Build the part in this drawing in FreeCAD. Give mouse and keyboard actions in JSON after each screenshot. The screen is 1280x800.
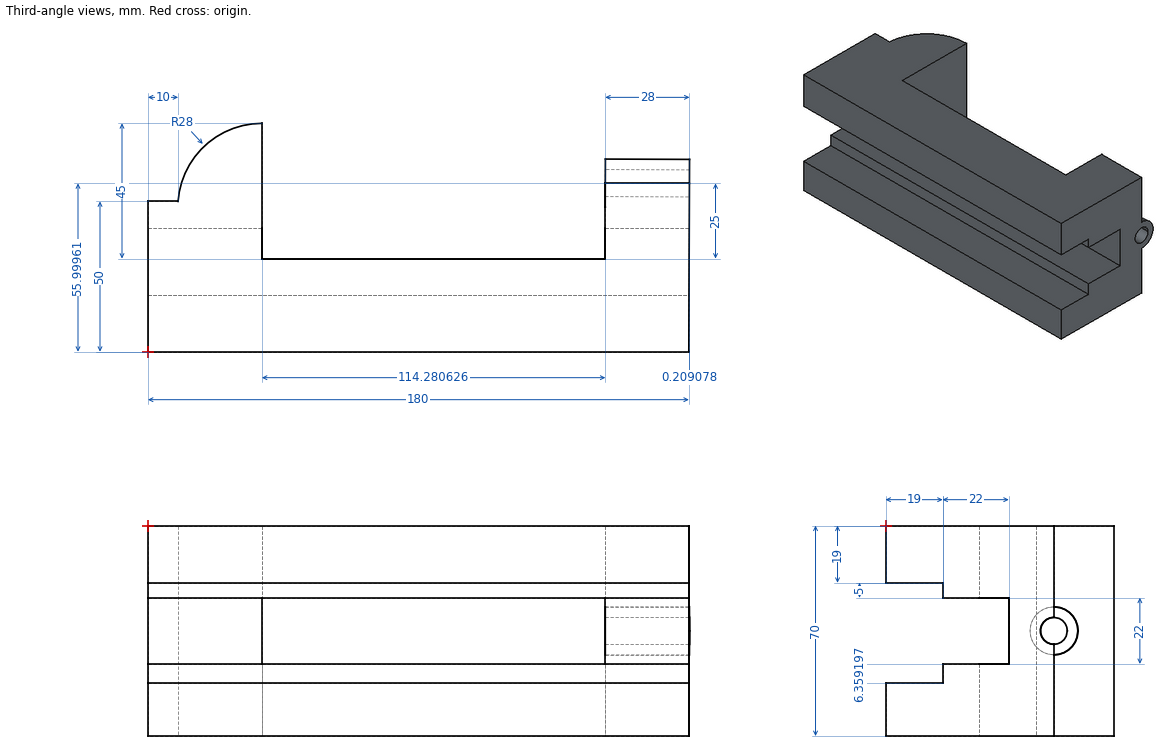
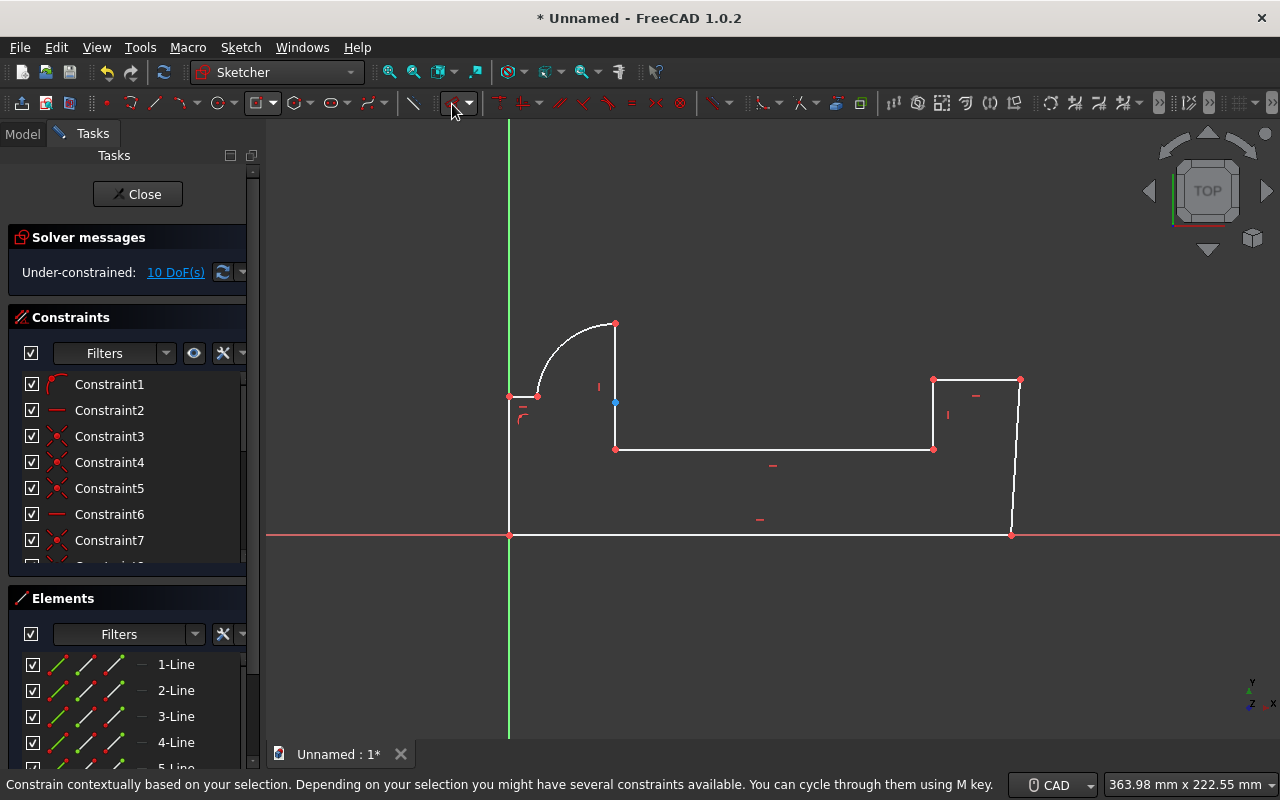
{"action": "left_click", "coordinate": [581, 332]}
{"action": "left_click", "coordinate": [567, 303]}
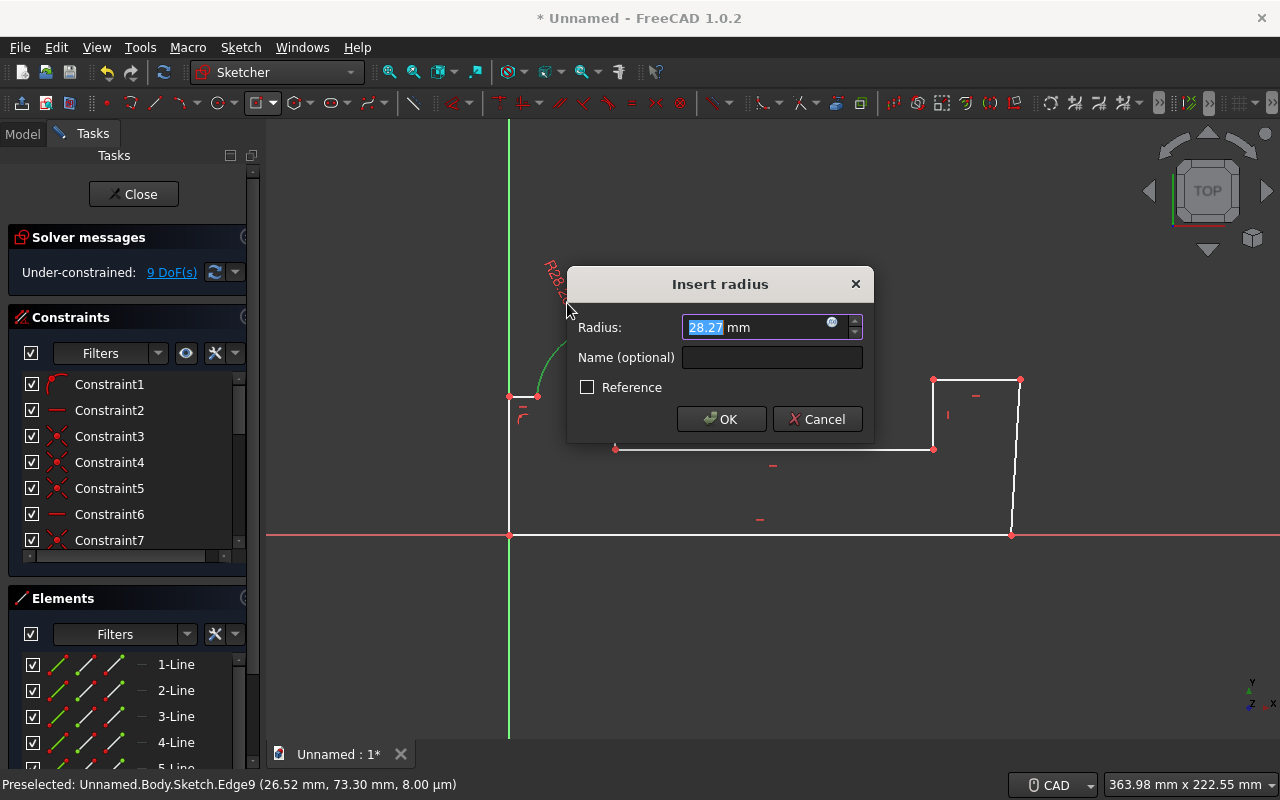
{"action": "type", "text": "28"}
{"action": "key", "text": "Return"}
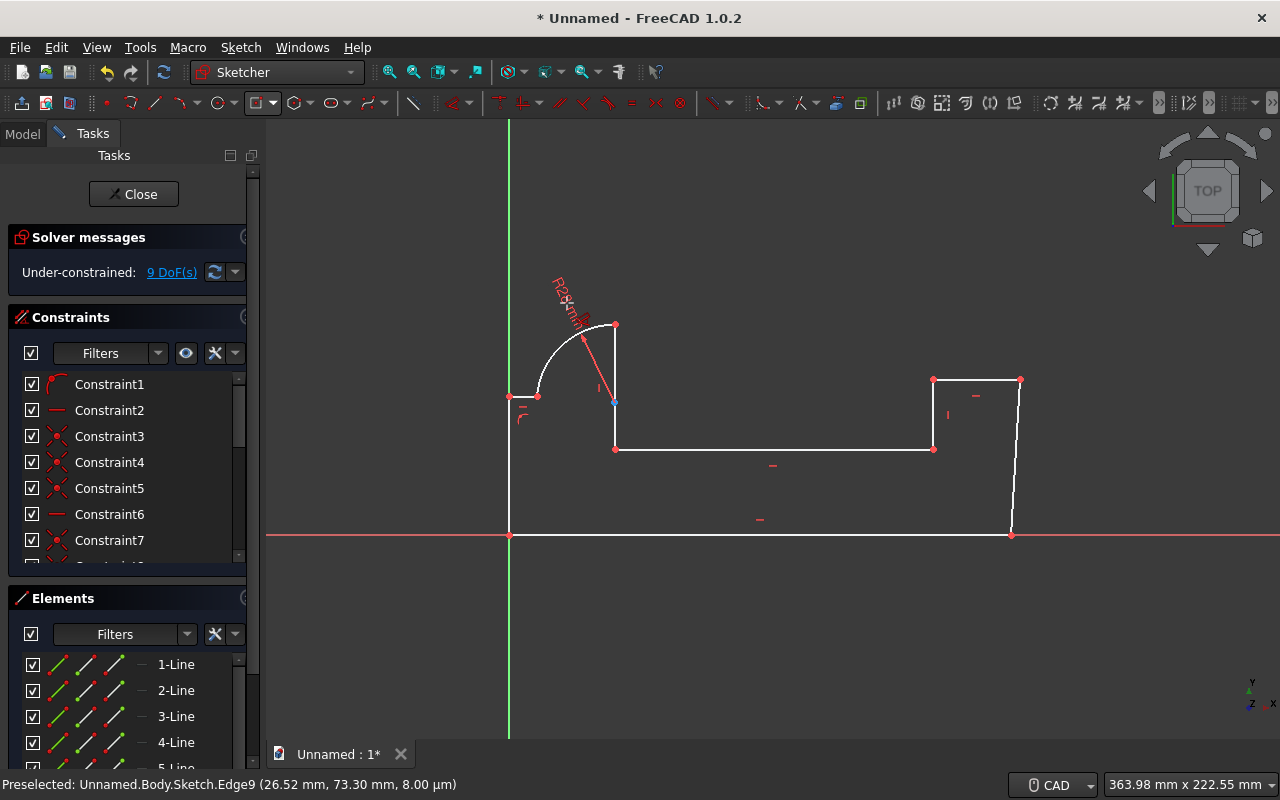
{"action": "scroll", "coordinate": [526, 397], "scroll_direction": "up", "scroll_amount": 2}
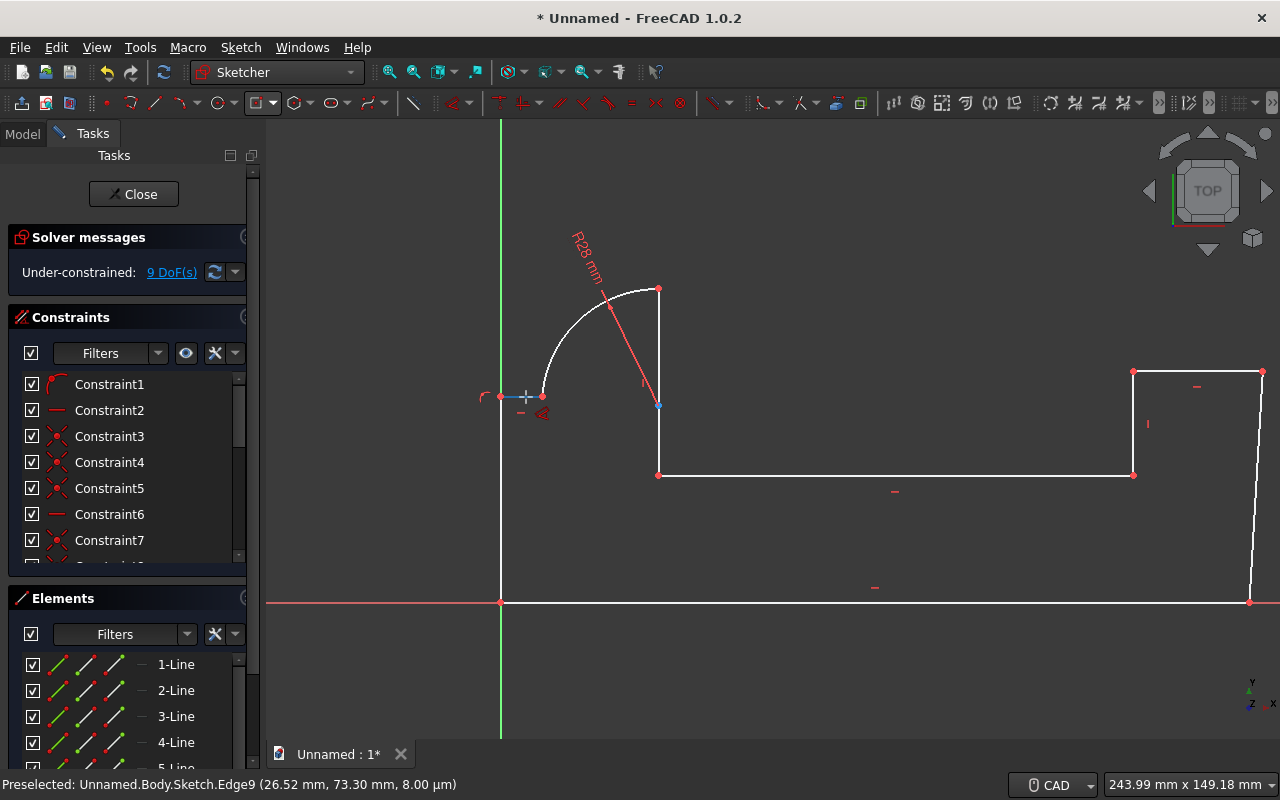
{"action": "left_click", "coordinate": [526, 397]}
{"action": "left_click", "coordinate": [522, 363]}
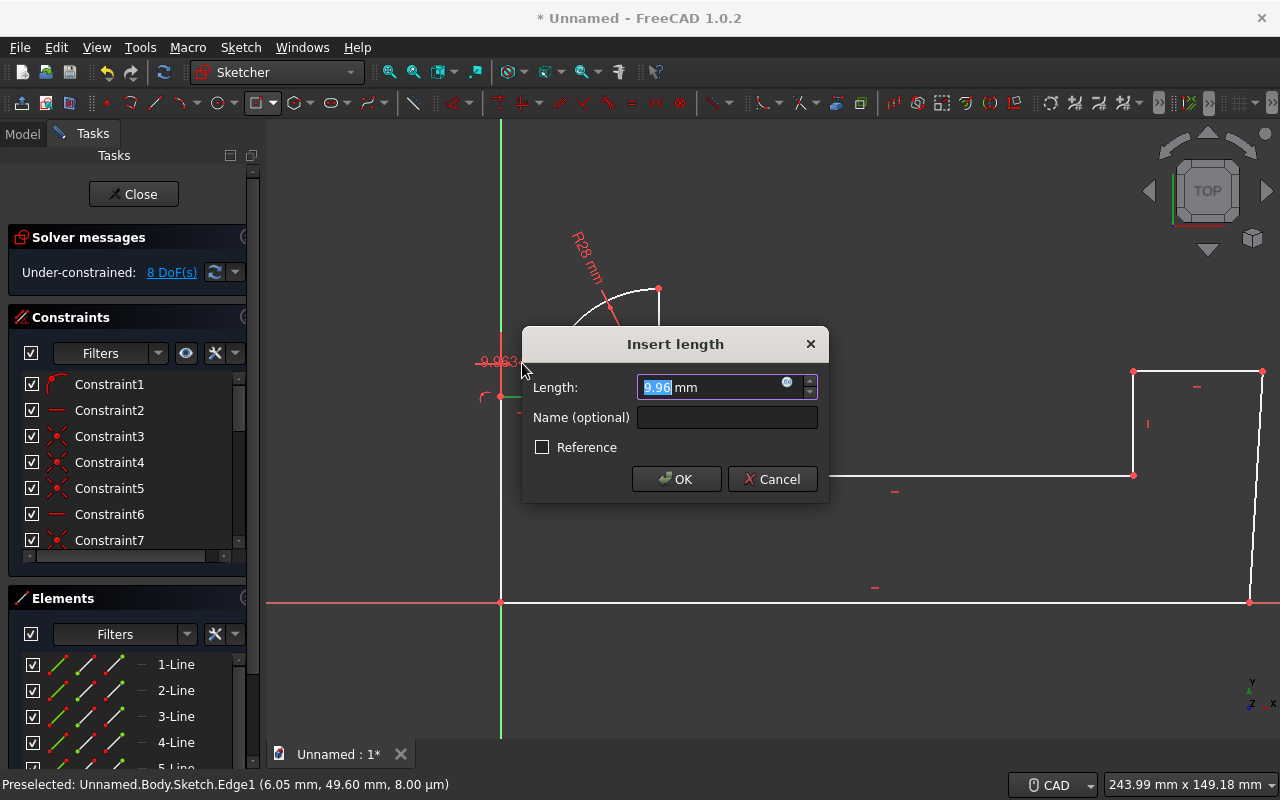
{"action": "type", "text": "10"}
{"action": "key", "text": "Return"}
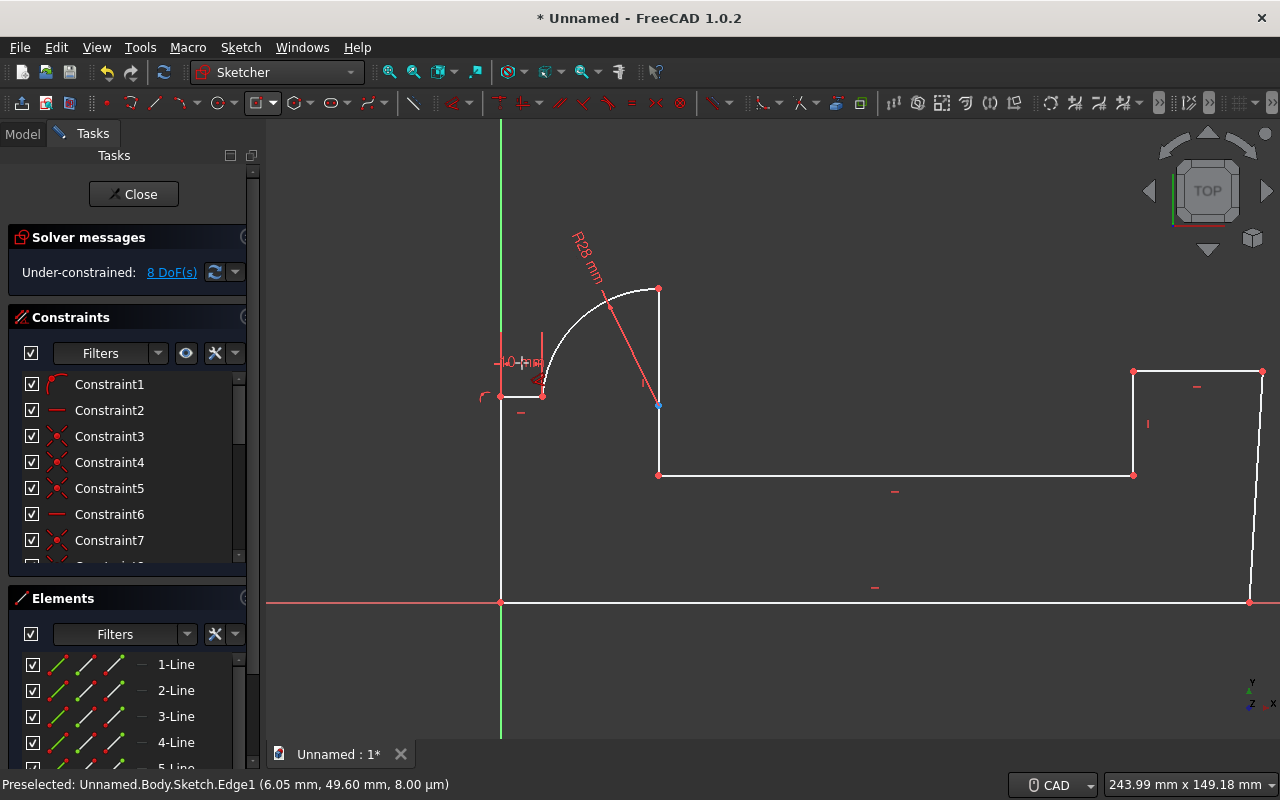
{"action": "left_click", "coordinate": [501, 459]}
{"action": "left_click", "coordinate": [467, 500]}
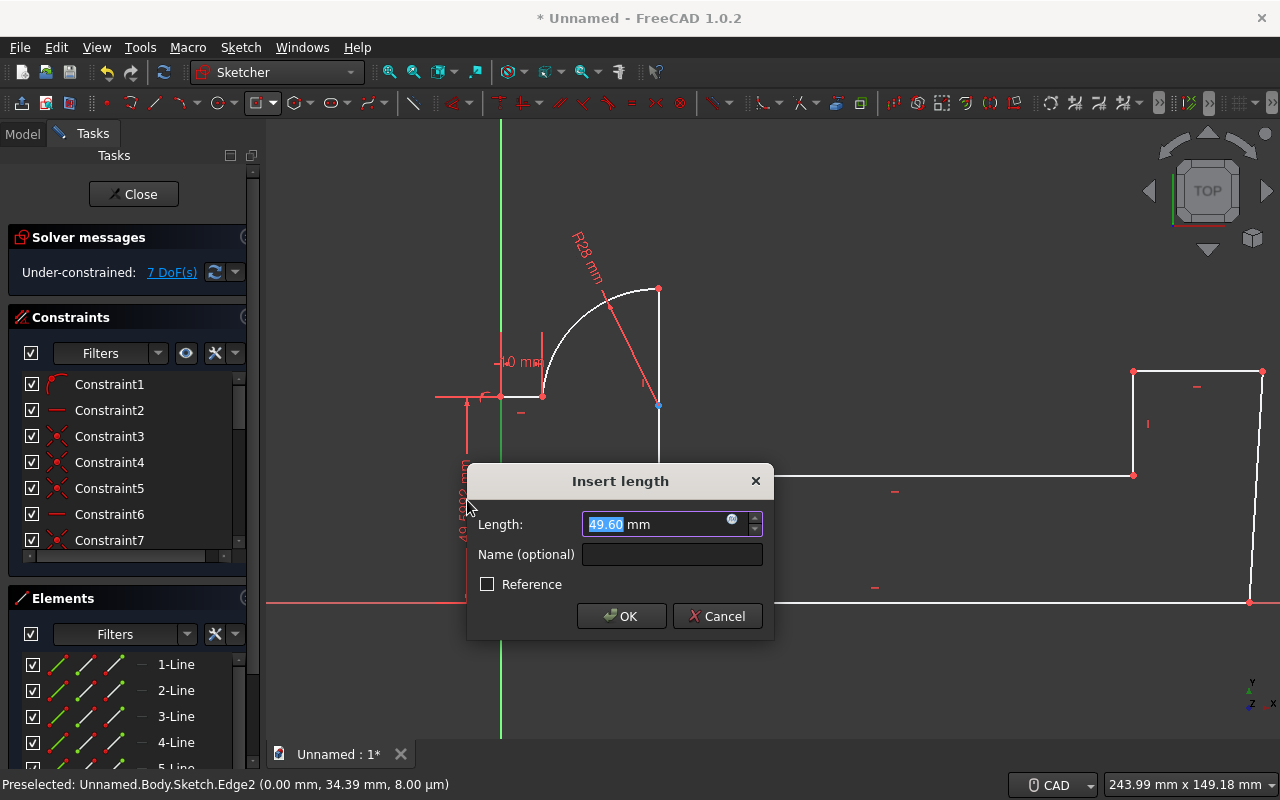
{"action": "type", "text": "50"}
{"action": "key", "text": "Return"}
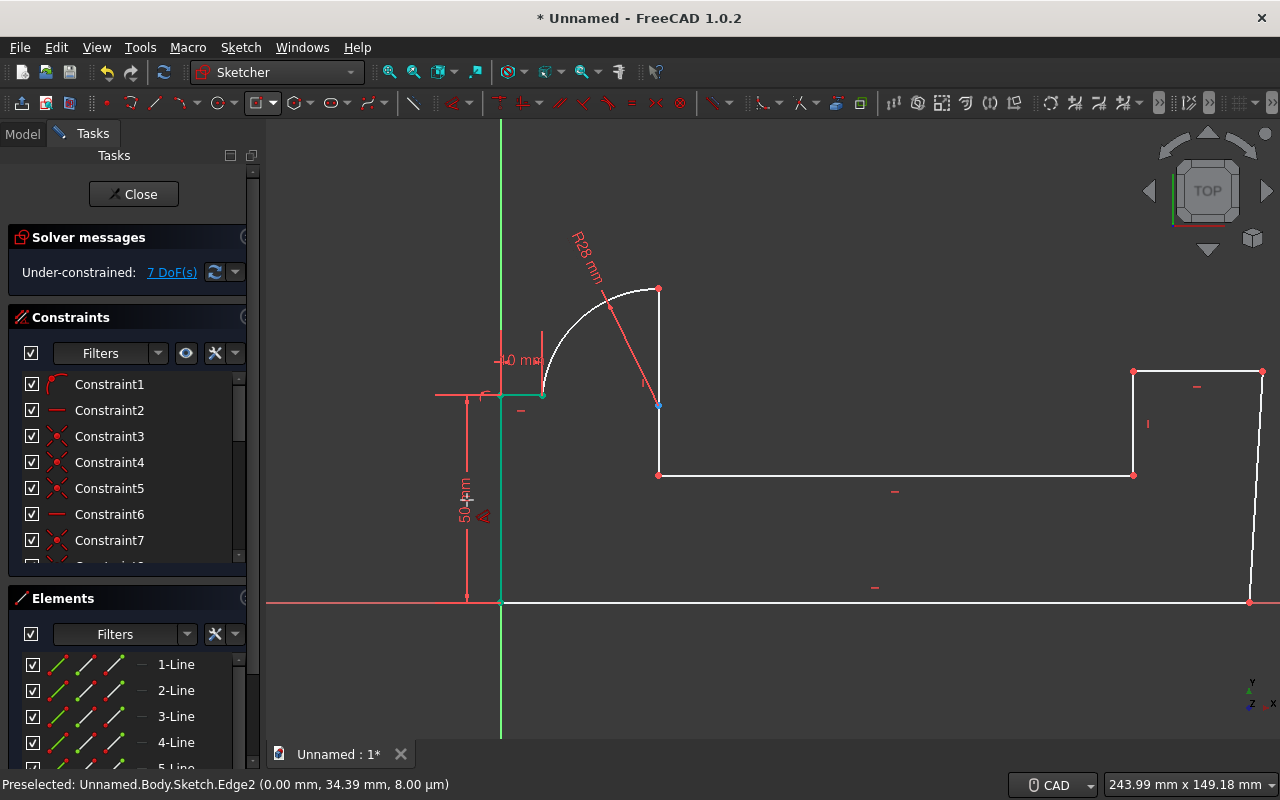
{"action": "scroll", "coordinate": [294, 357], "scroll_direction": "down", "scroll_amount": 1}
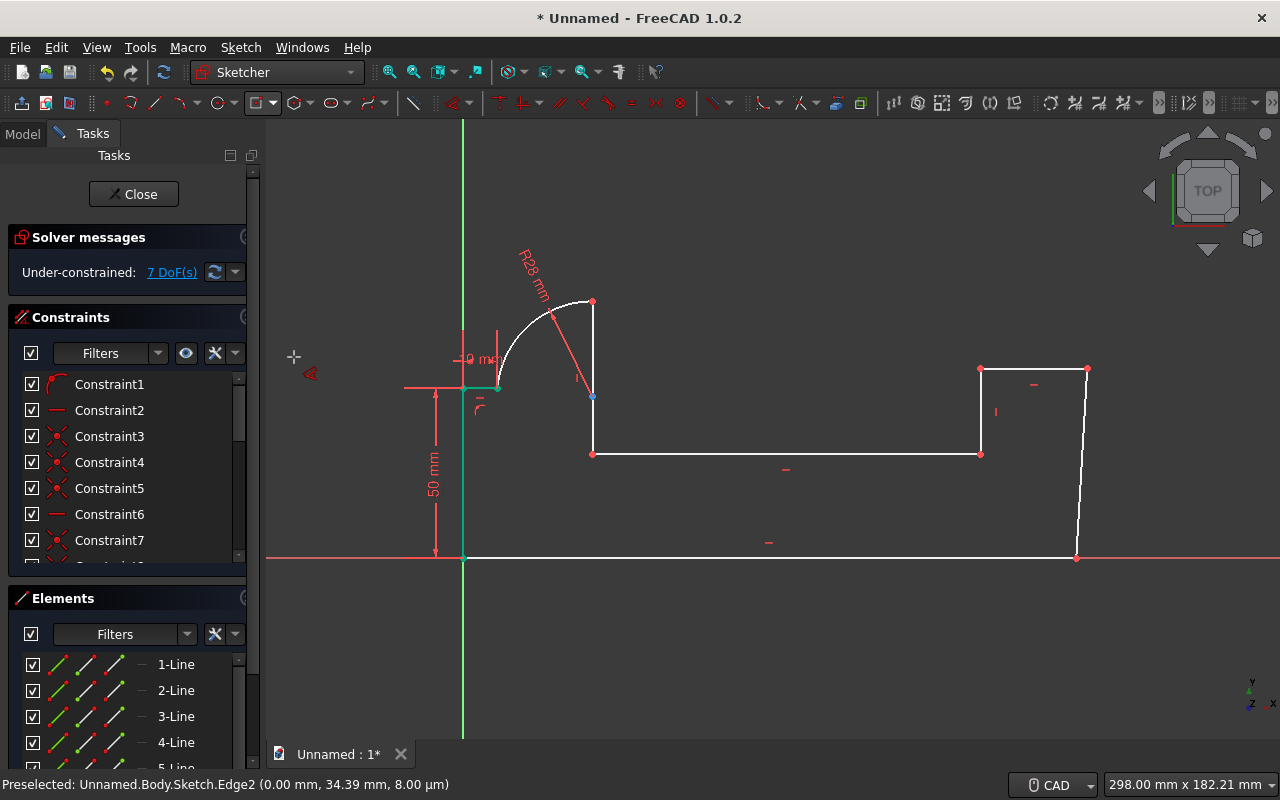
{"action": "left_click", "coordinate": [1055, 369]}
{"action": "left_click", "coordinate": [1034, 335]}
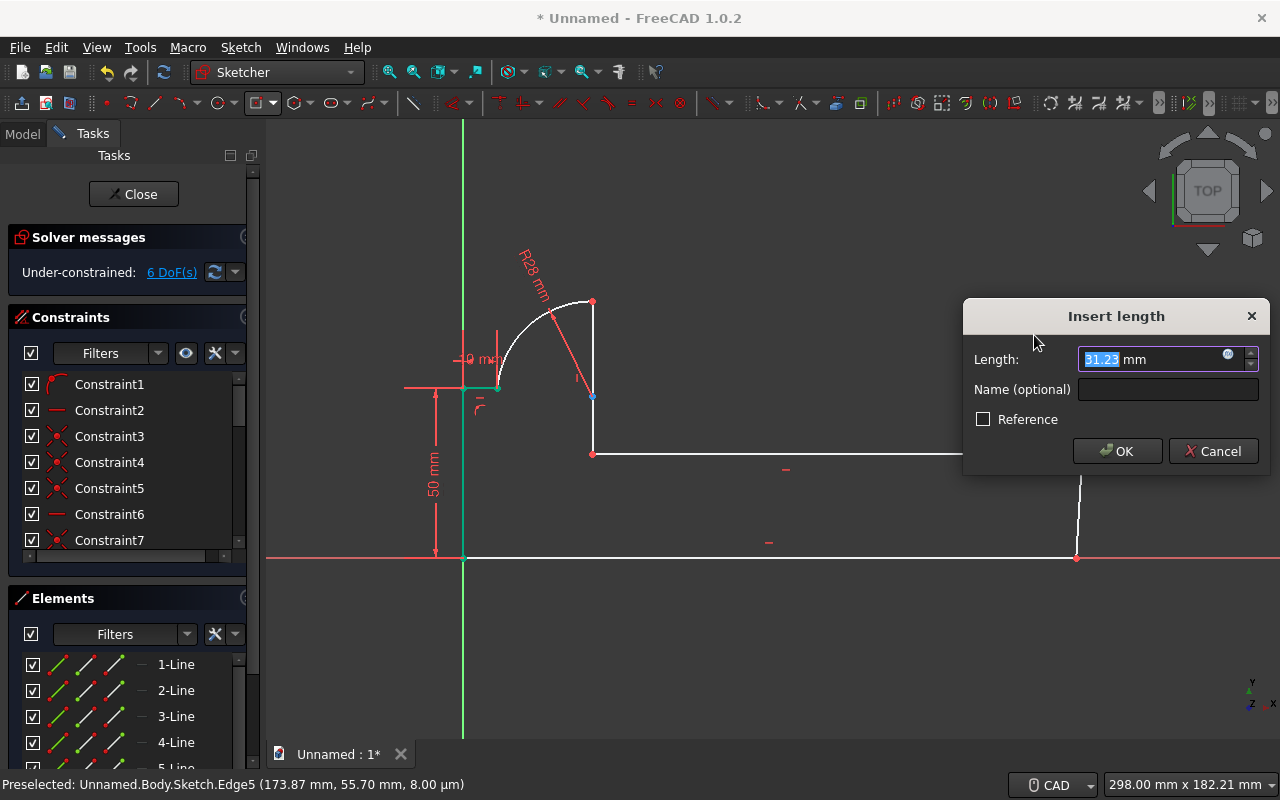
{"action": "type", "text": "28"}
{"action": "key", "text": "Return"}